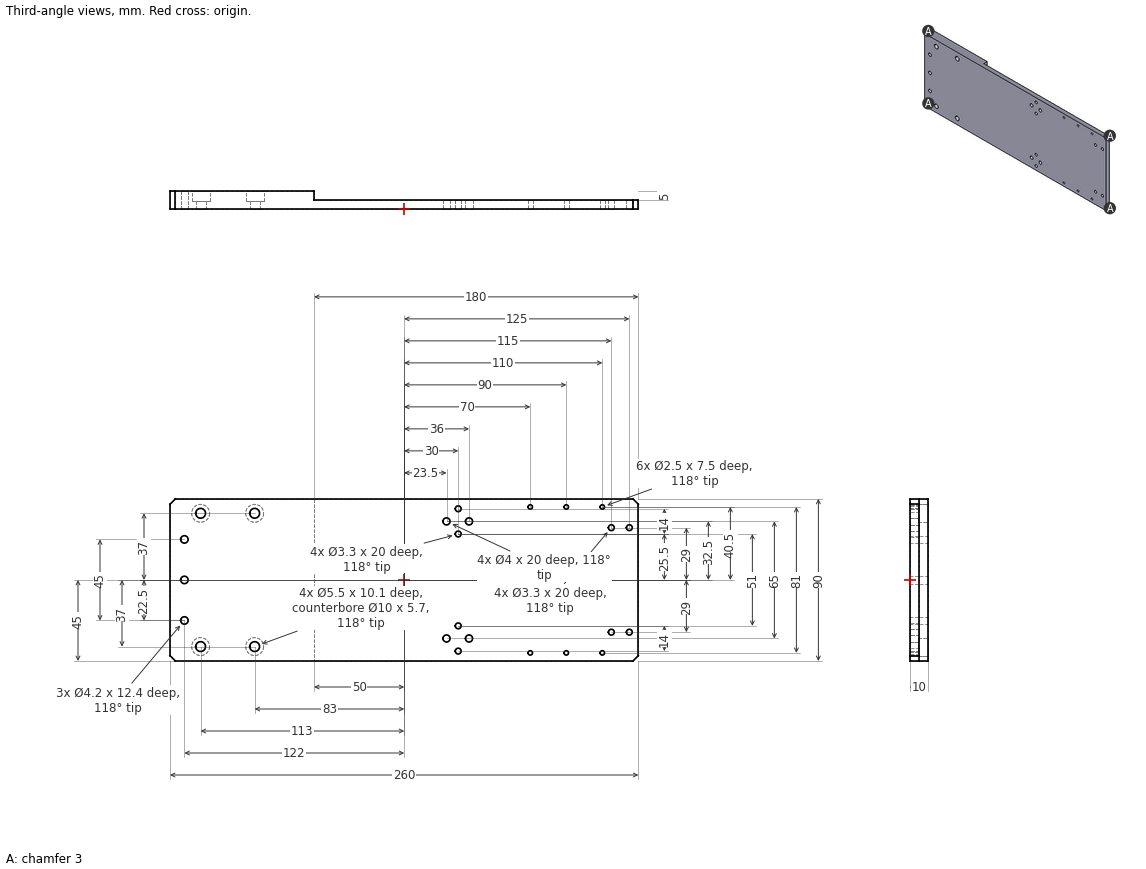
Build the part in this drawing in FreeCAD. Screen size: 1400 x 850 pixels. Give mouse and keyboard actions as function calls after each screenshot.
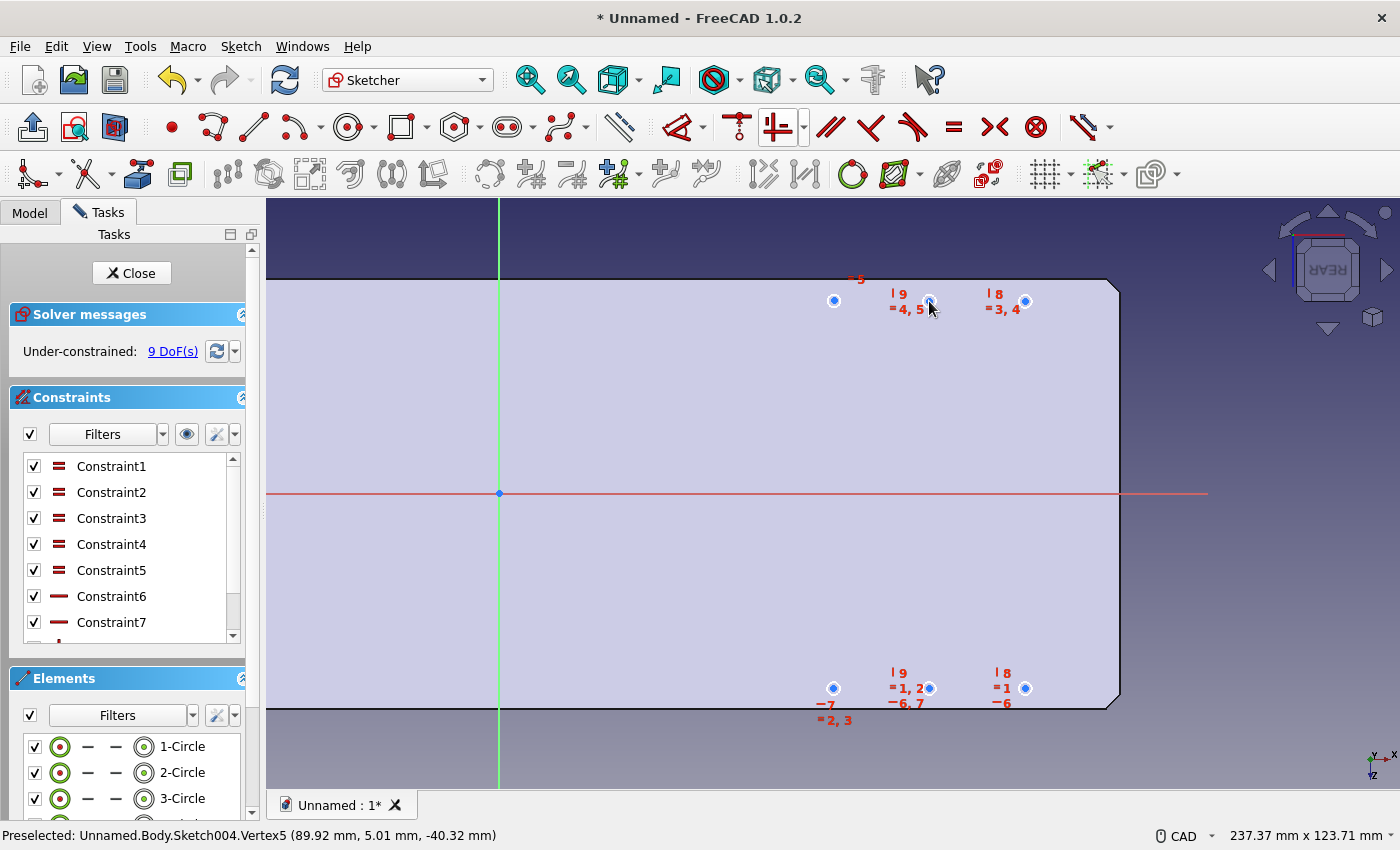
click(1025, 301)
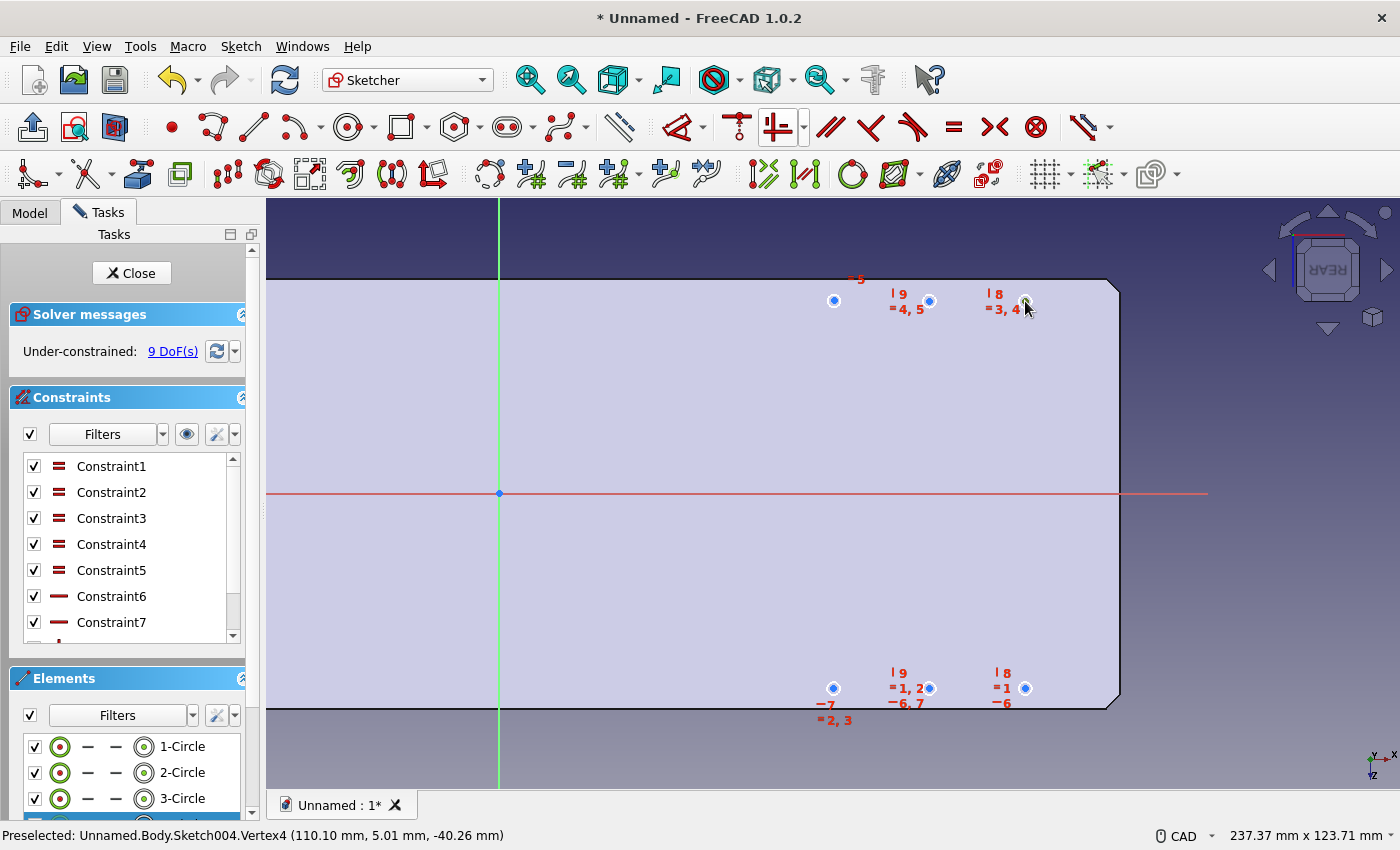
click(929, 301)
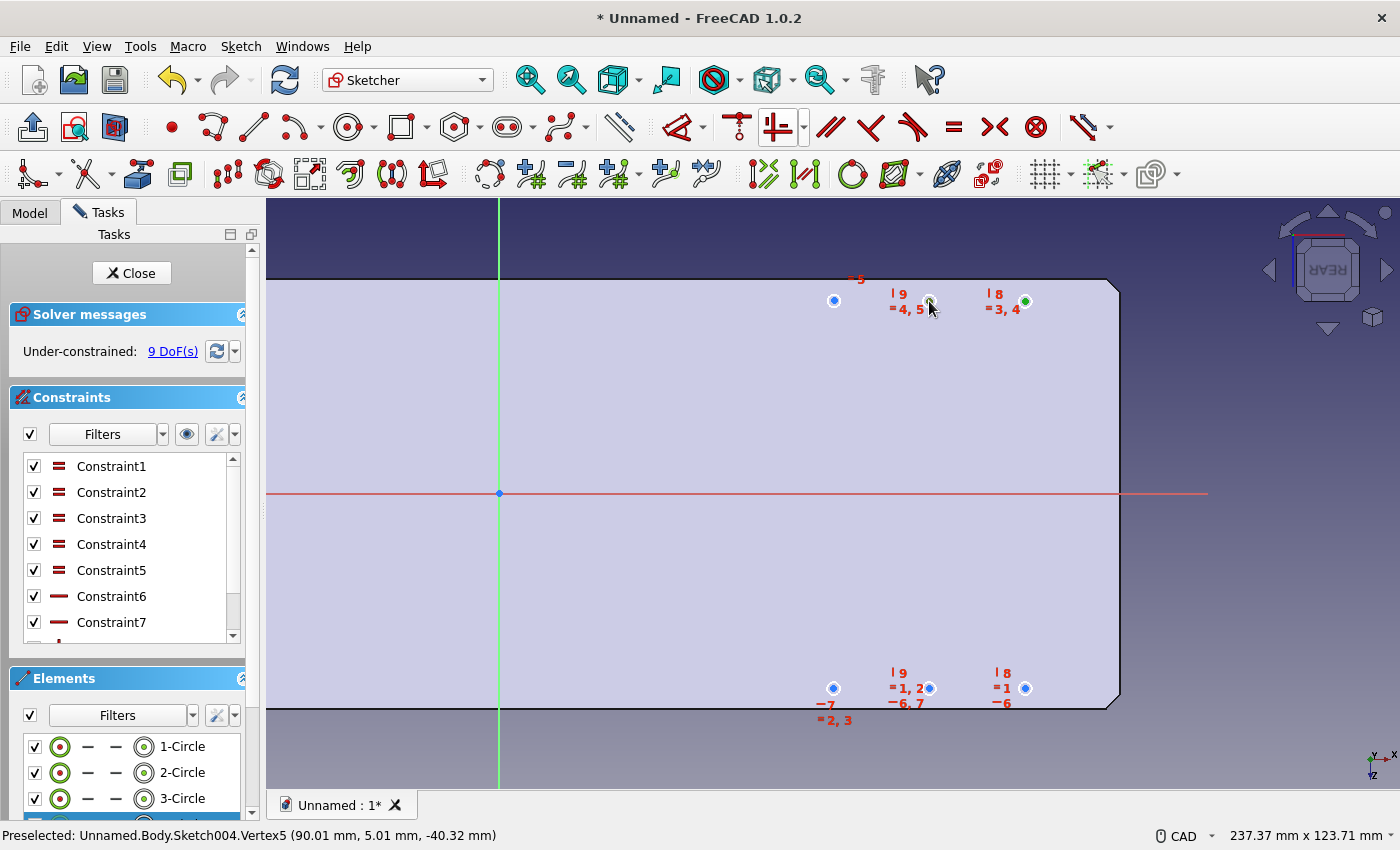
click(804, 128)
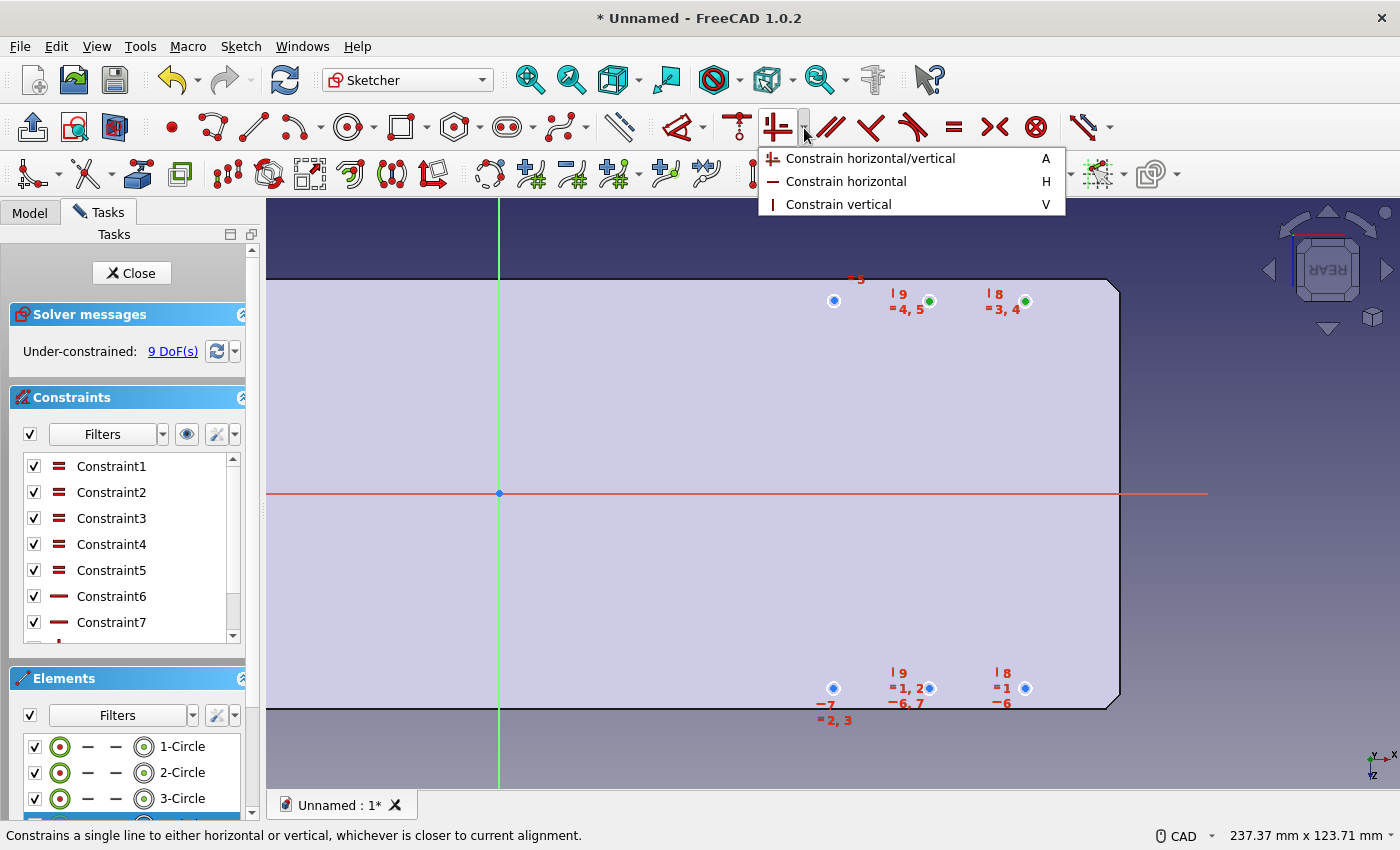
click(912, 182)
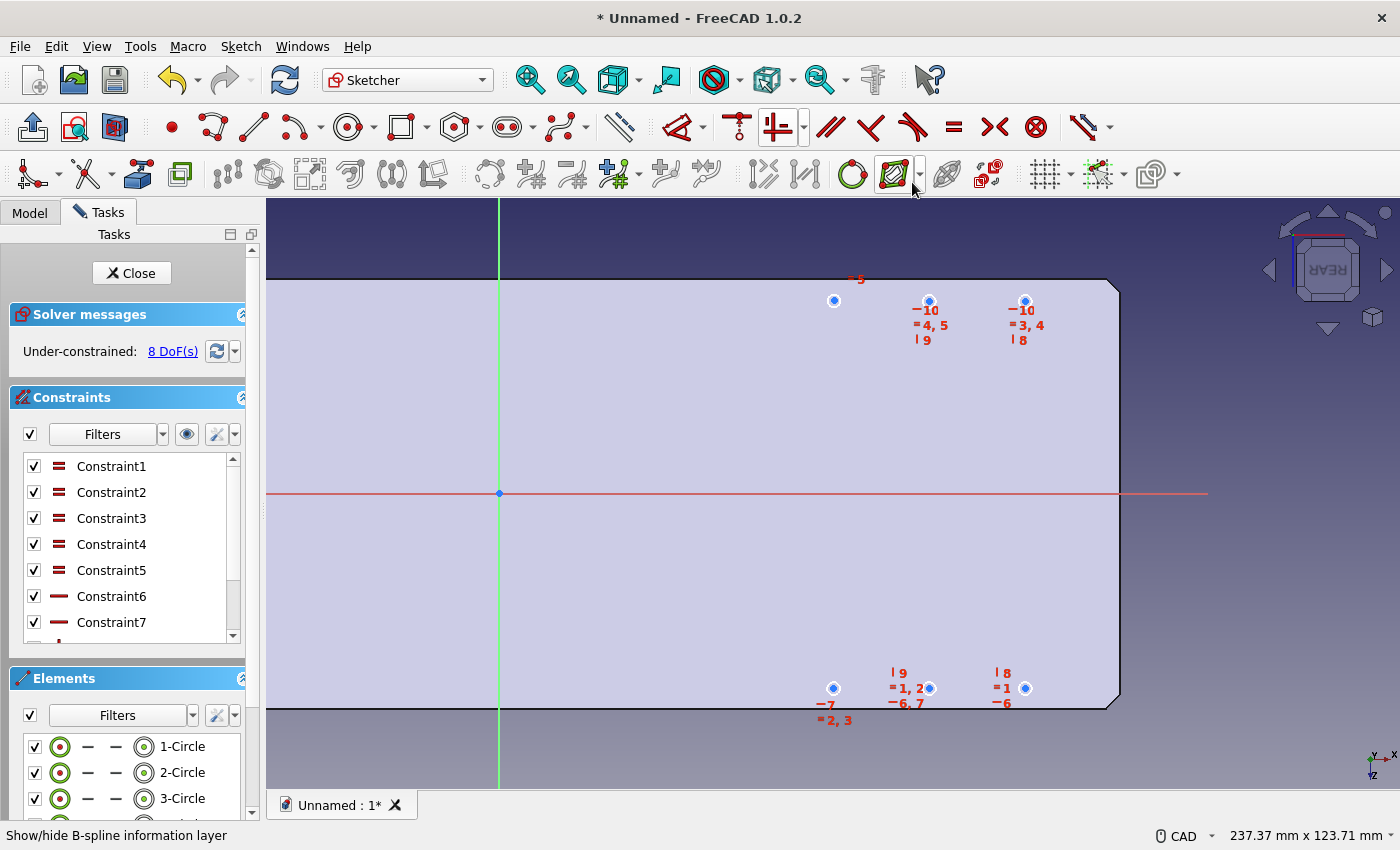
click(834, 689)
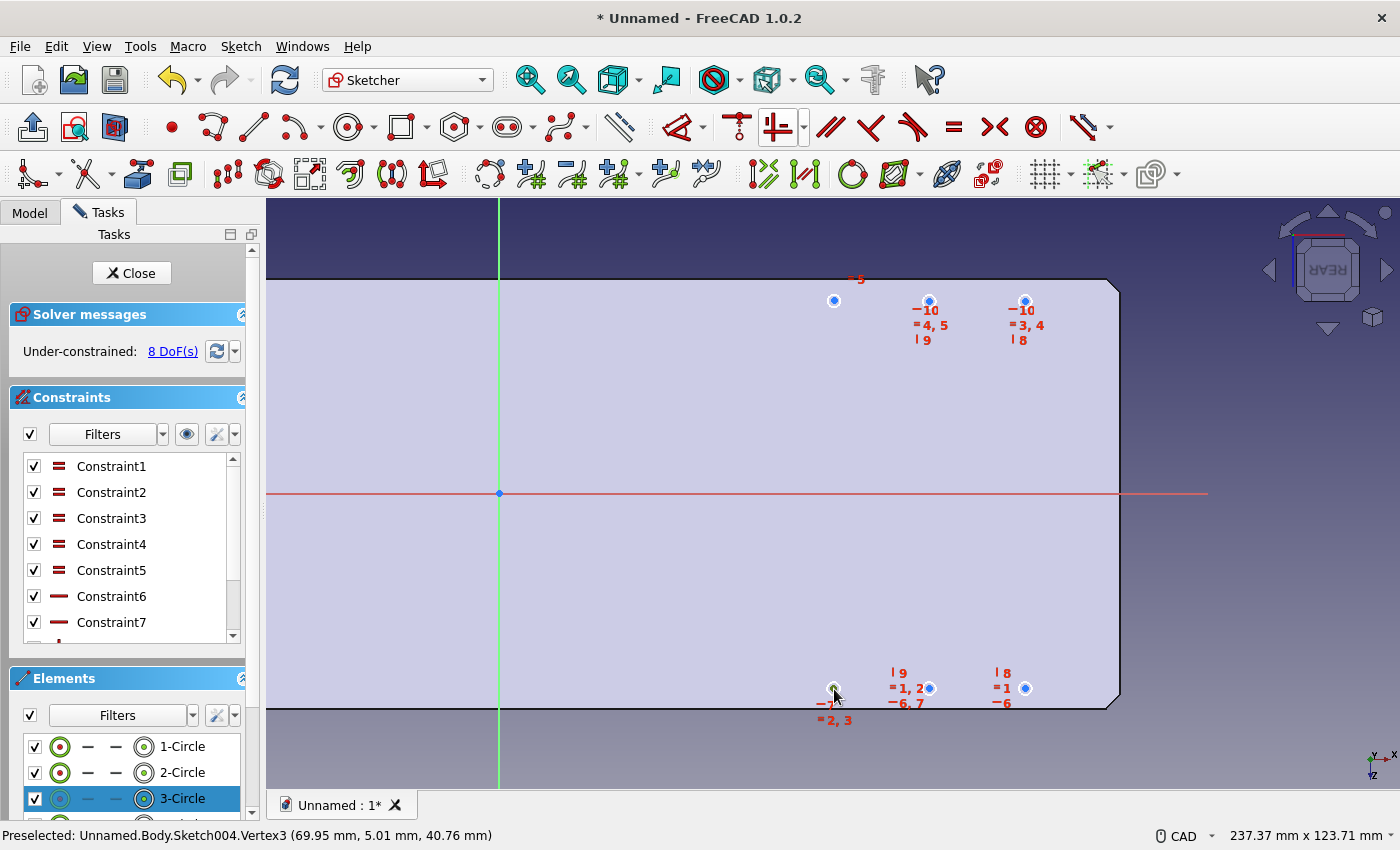
click(834, 301)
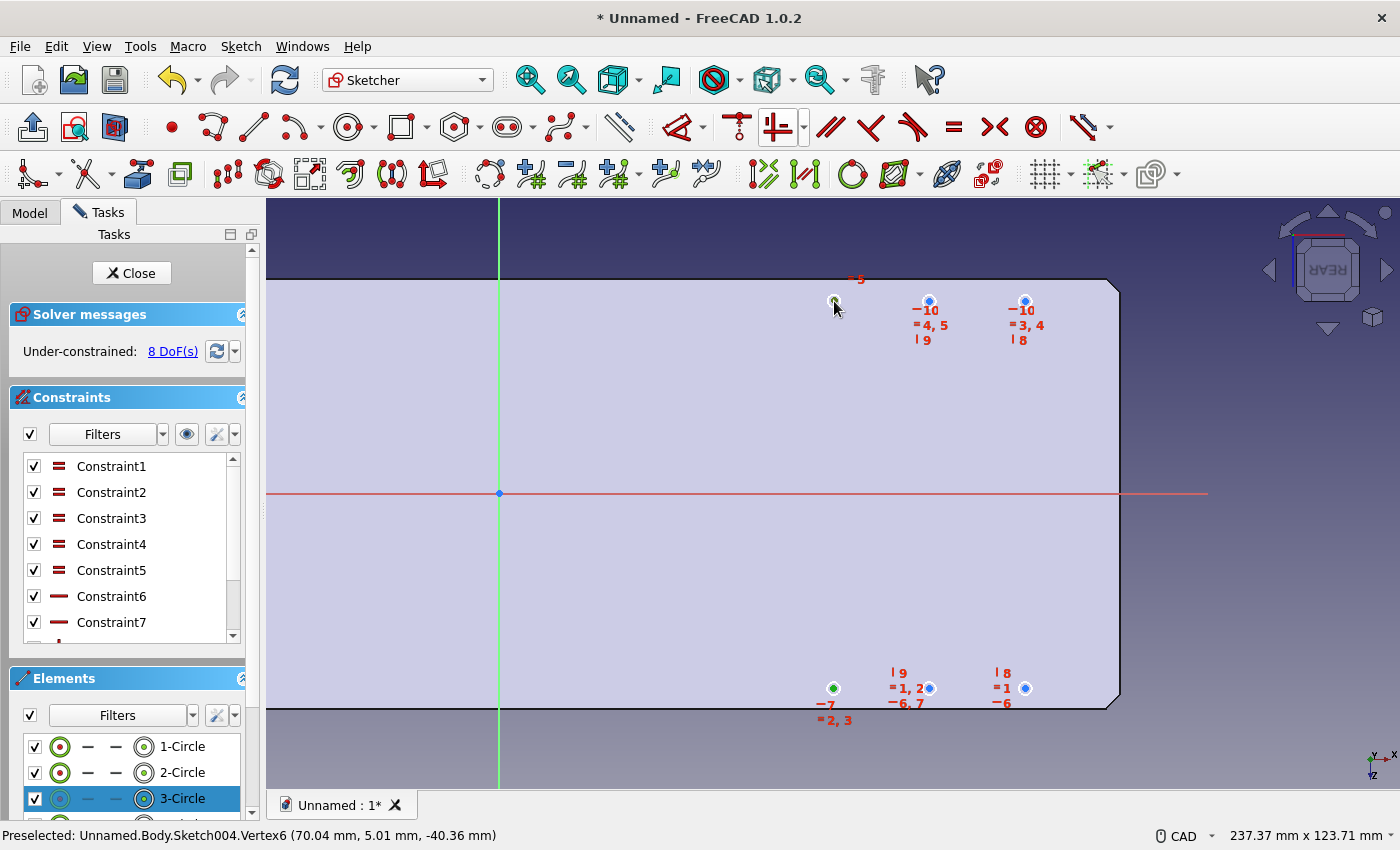
key(v)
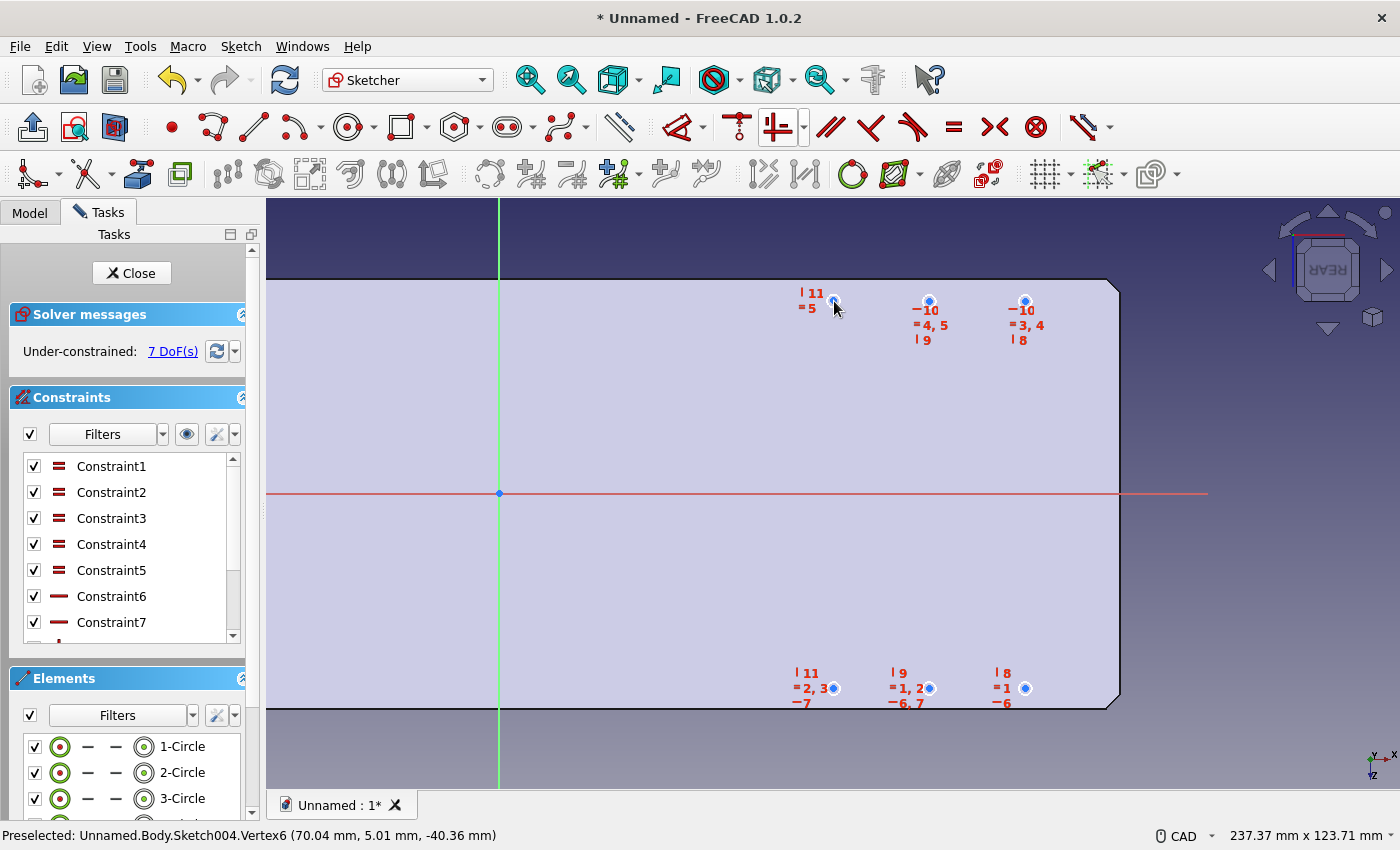
click(929, 301)